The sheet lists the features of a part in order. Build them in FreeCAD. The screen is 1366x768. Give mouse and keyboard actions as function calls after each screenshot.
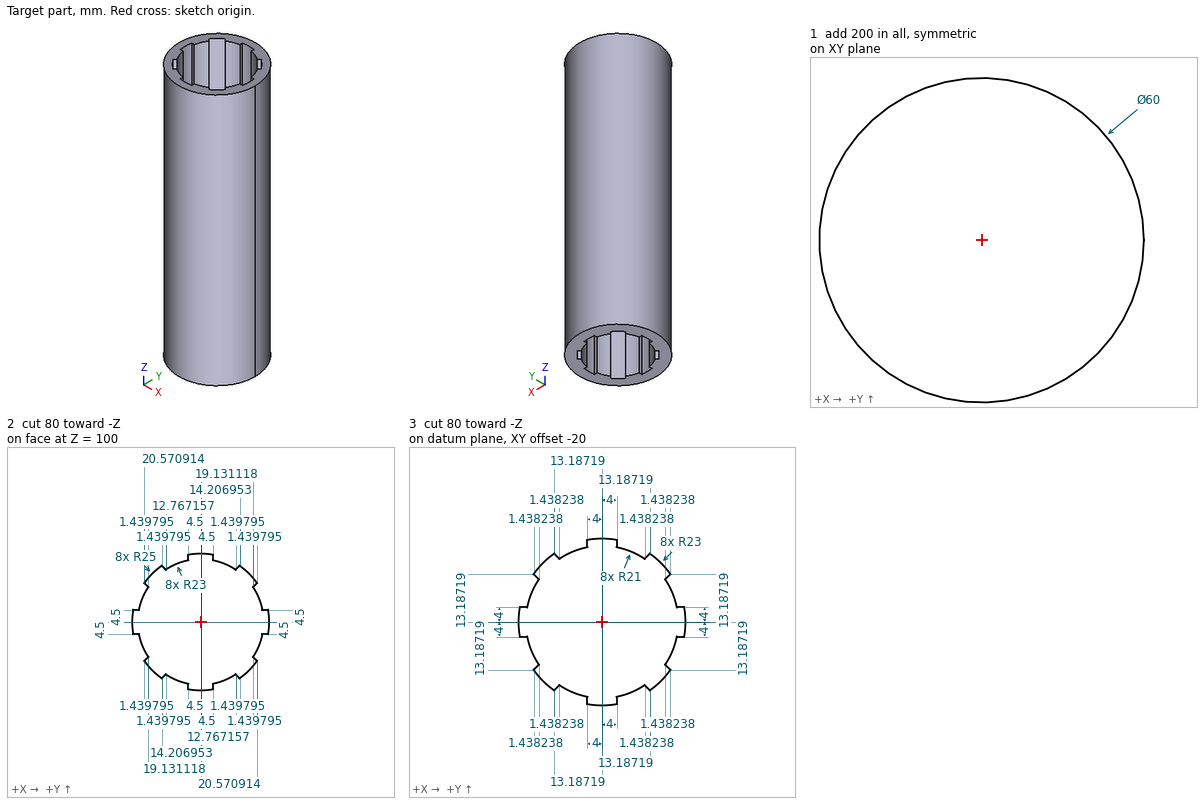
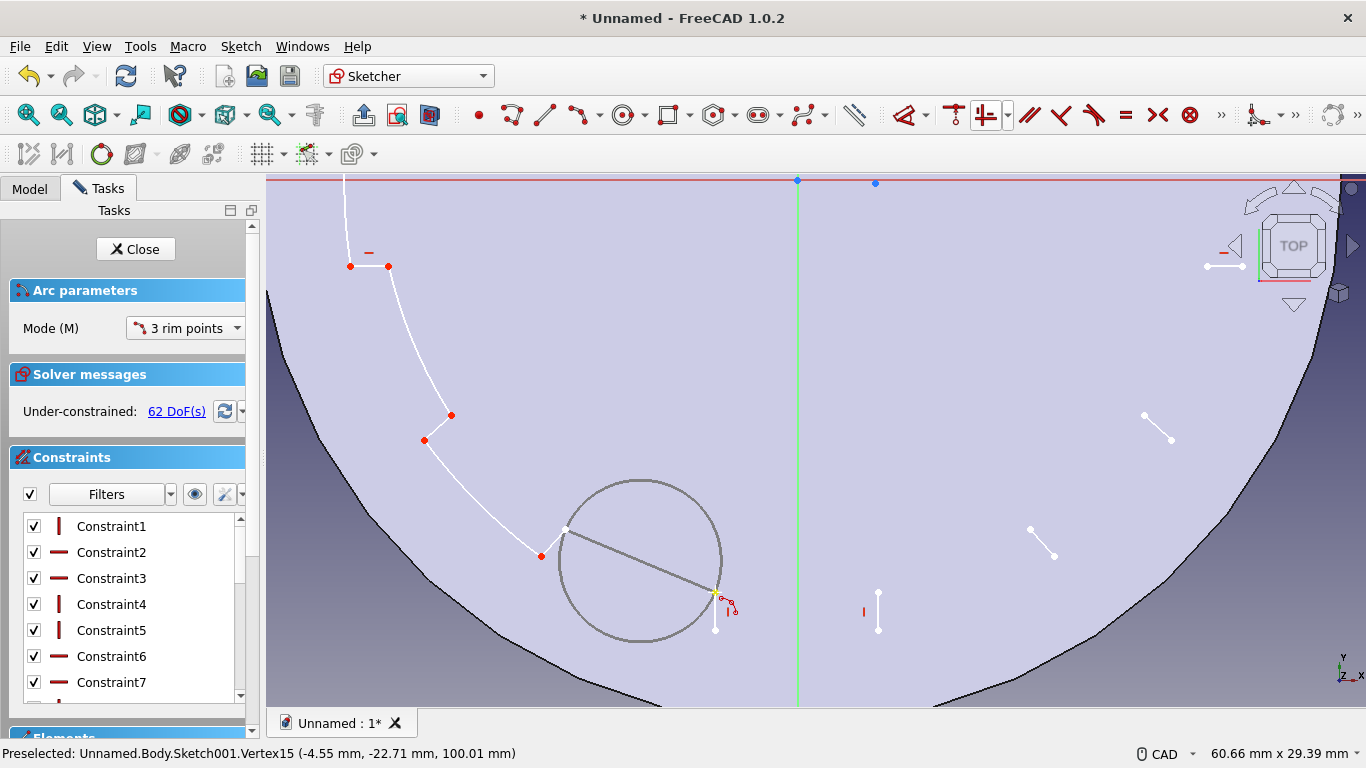
scroll(638, 566, up, 4)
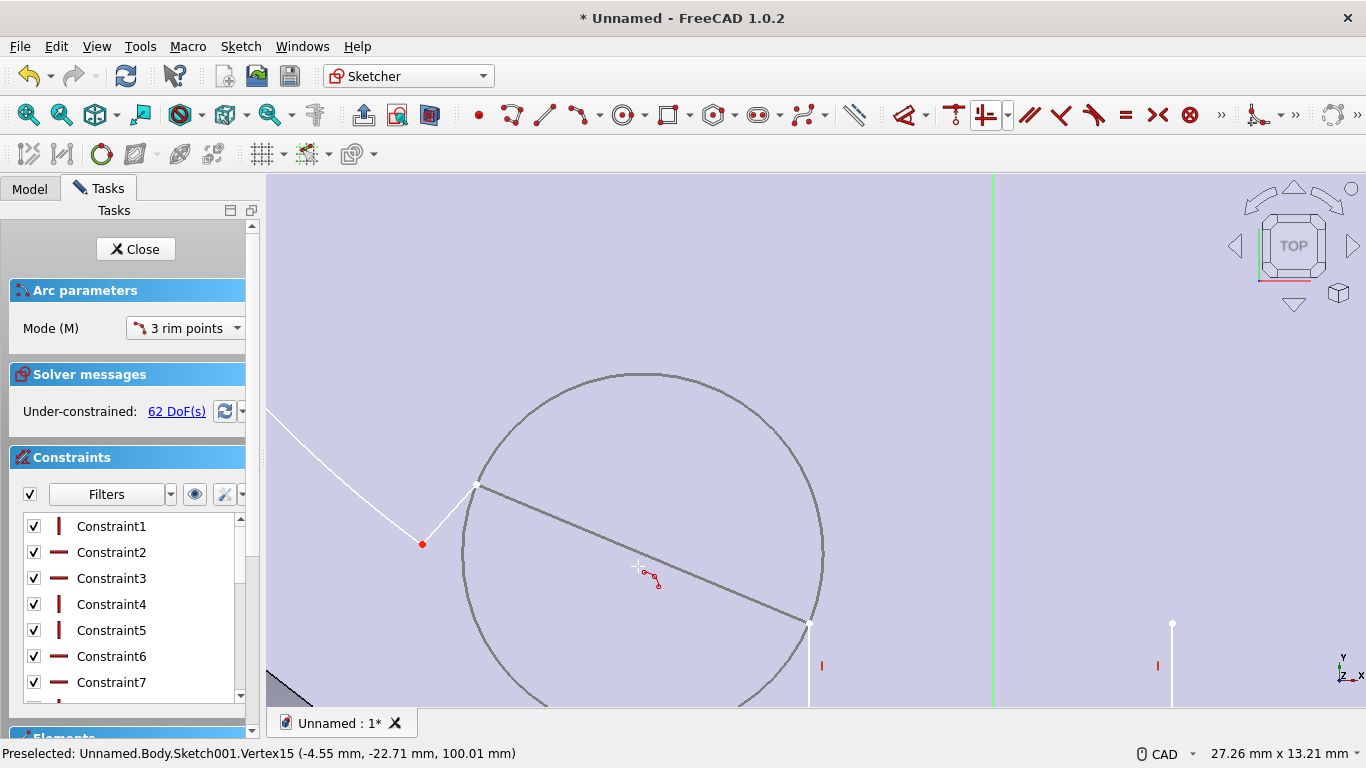
click(638, 565)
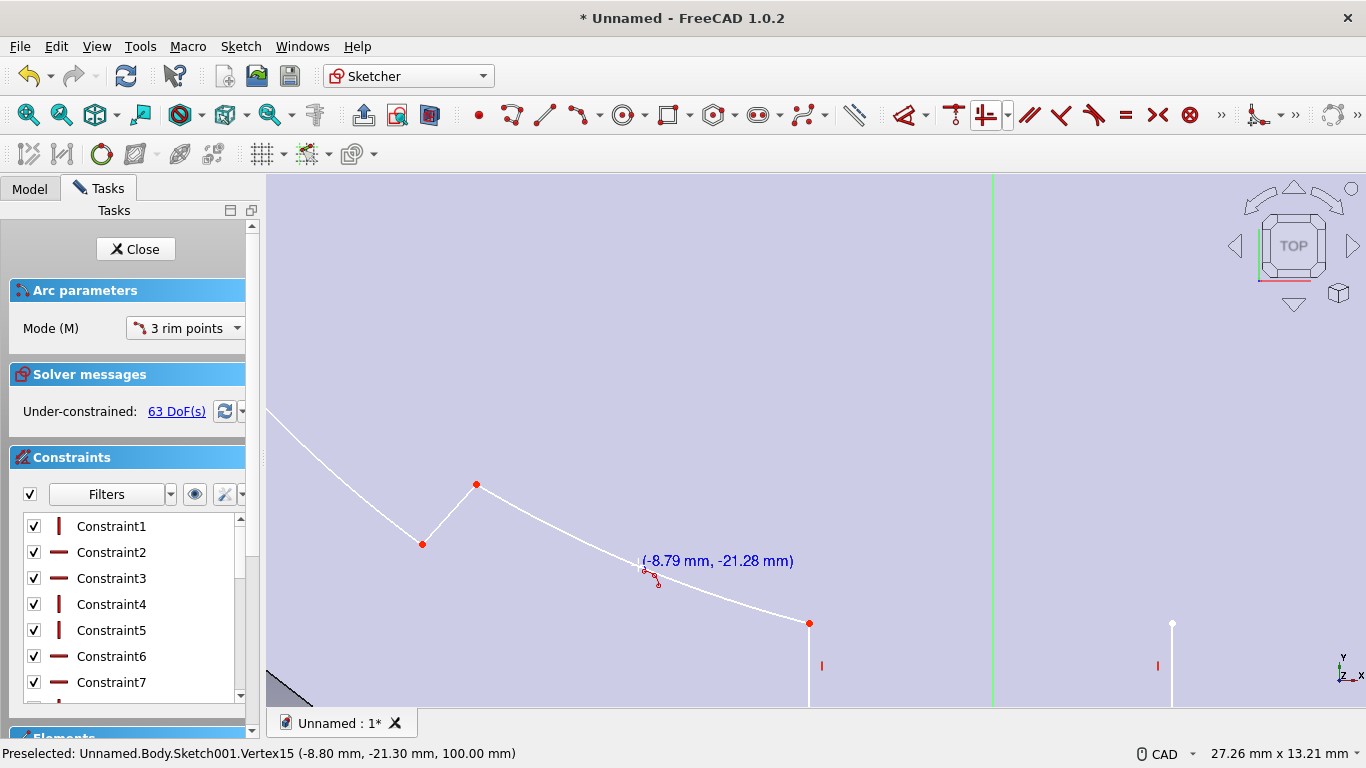
scroll(699, 586, down, 9)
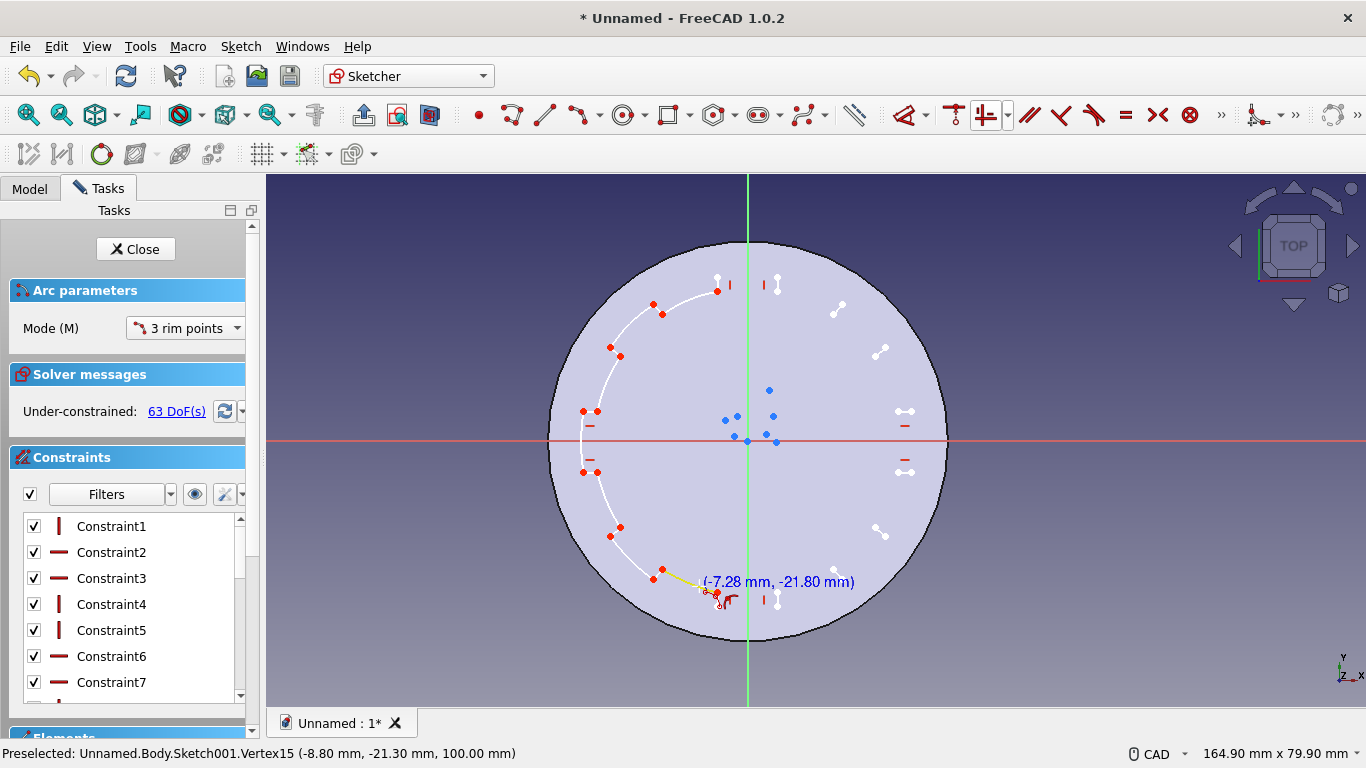
scroll(718, 605, up, 5)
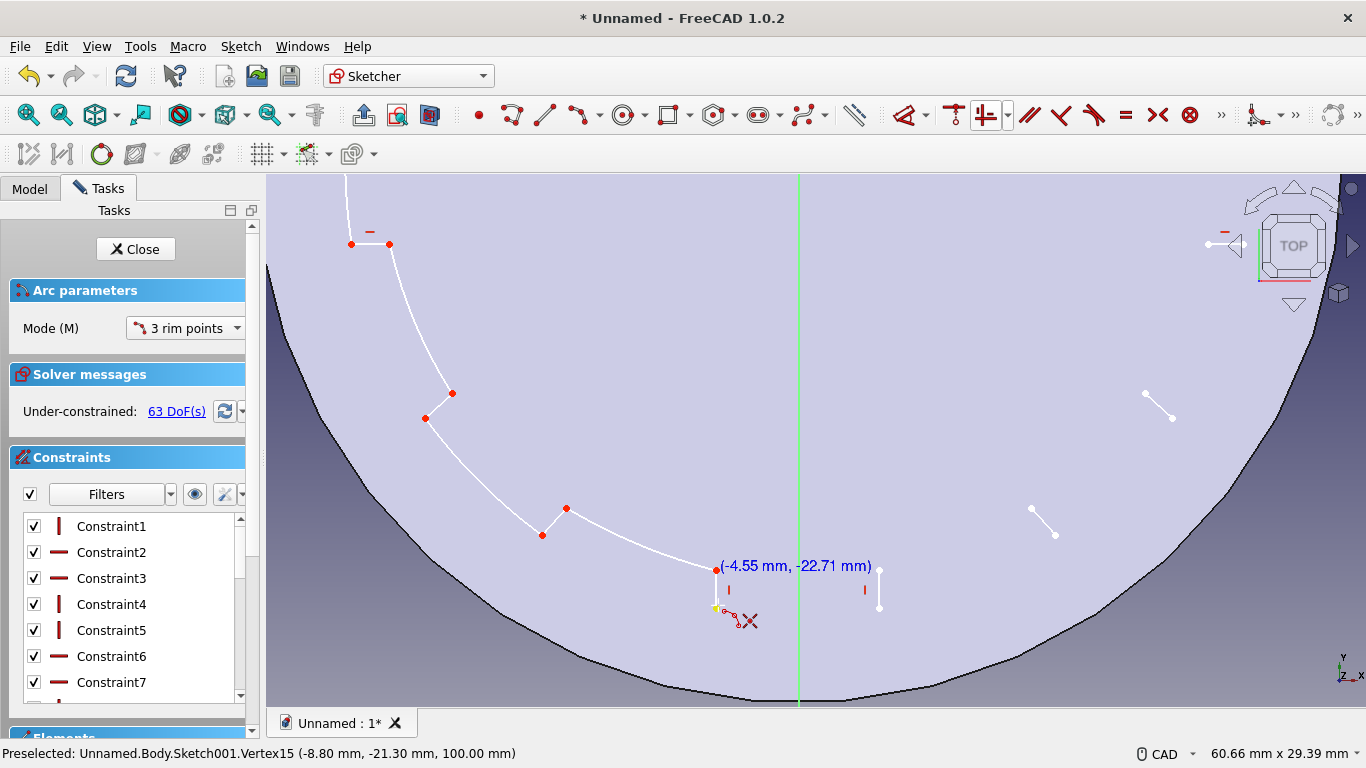
click(716, 609)
click(879, 609)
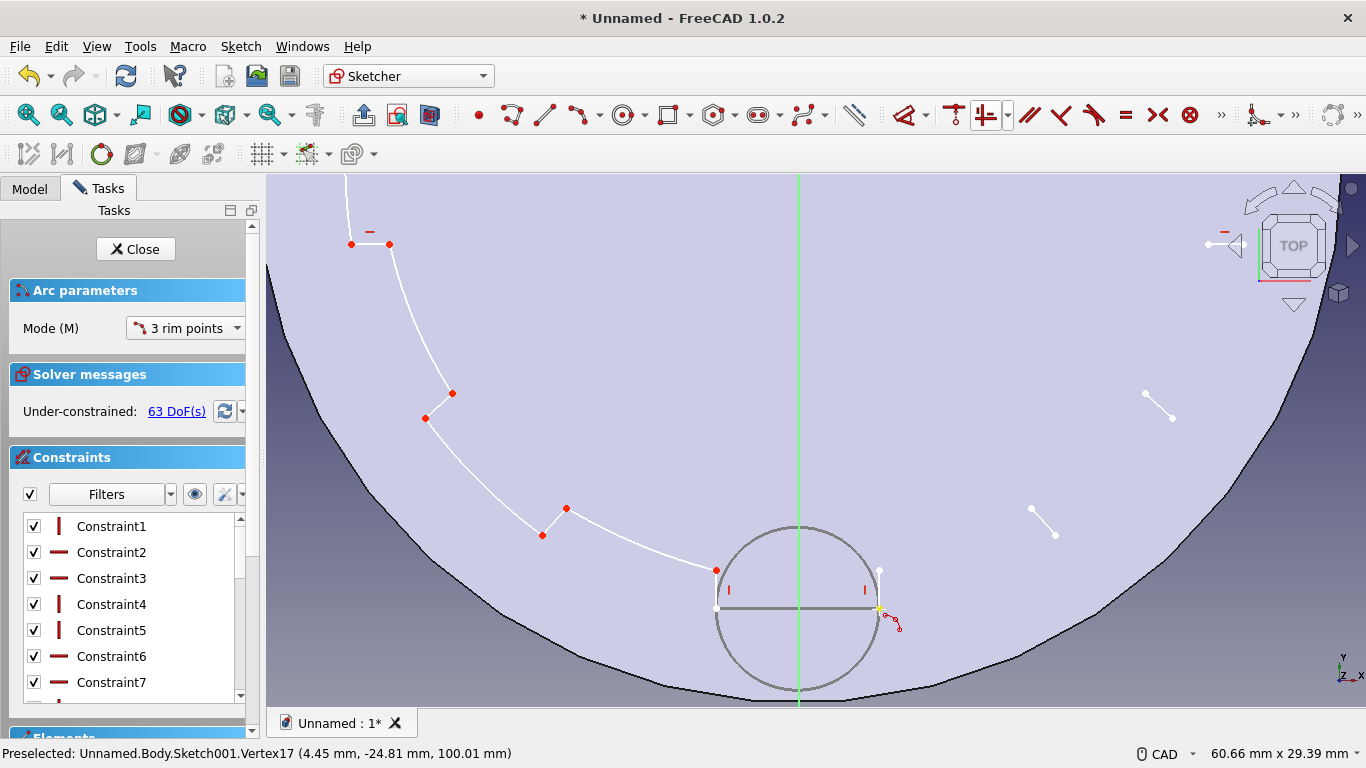
scroll(782, 612, up, 5)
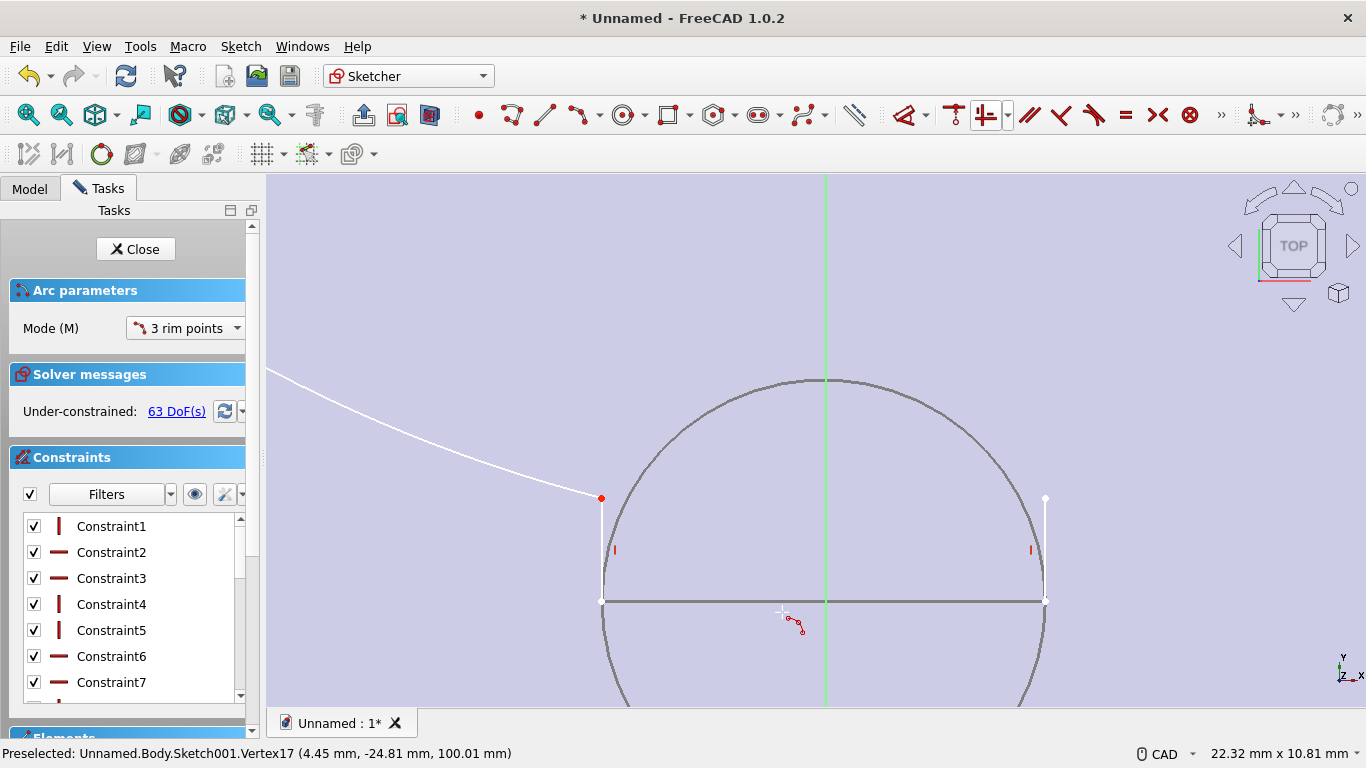
click(782, 610)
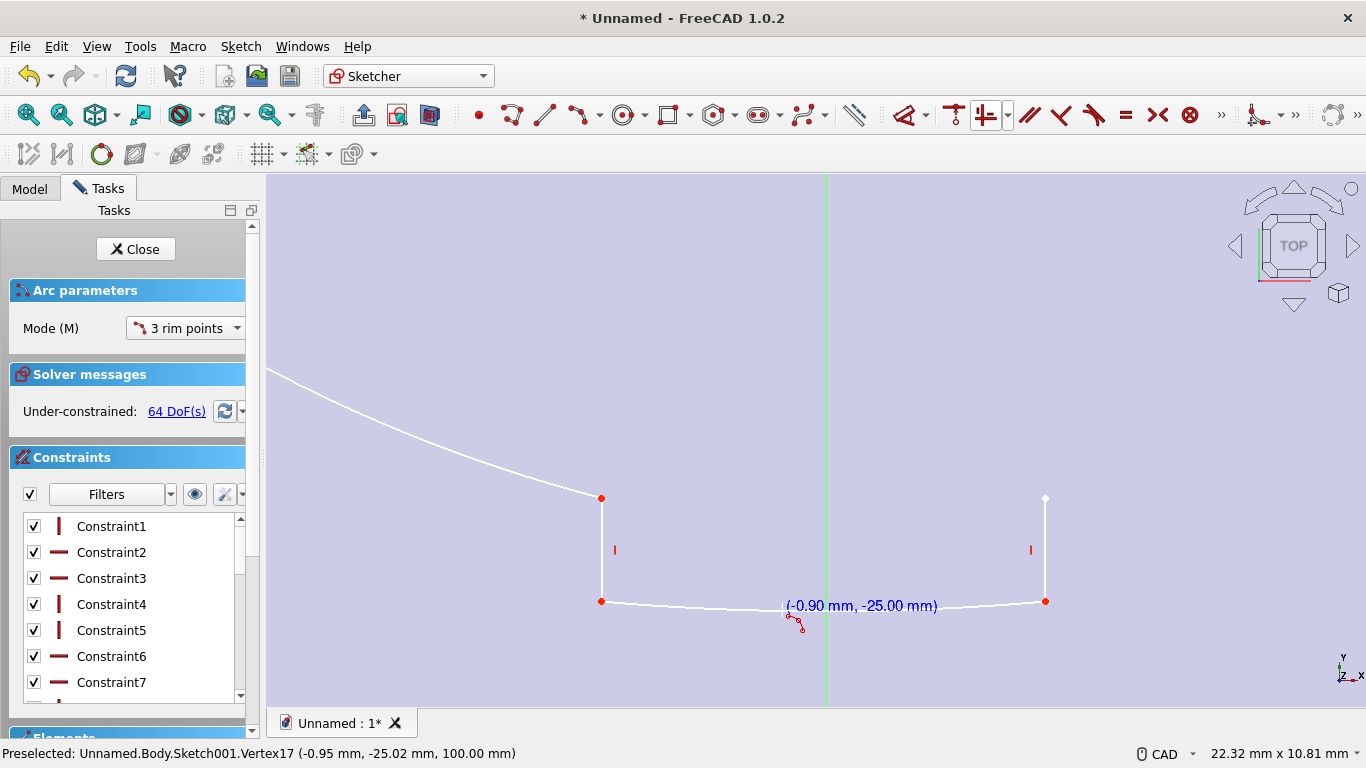
scroll(735, 607, down, 10)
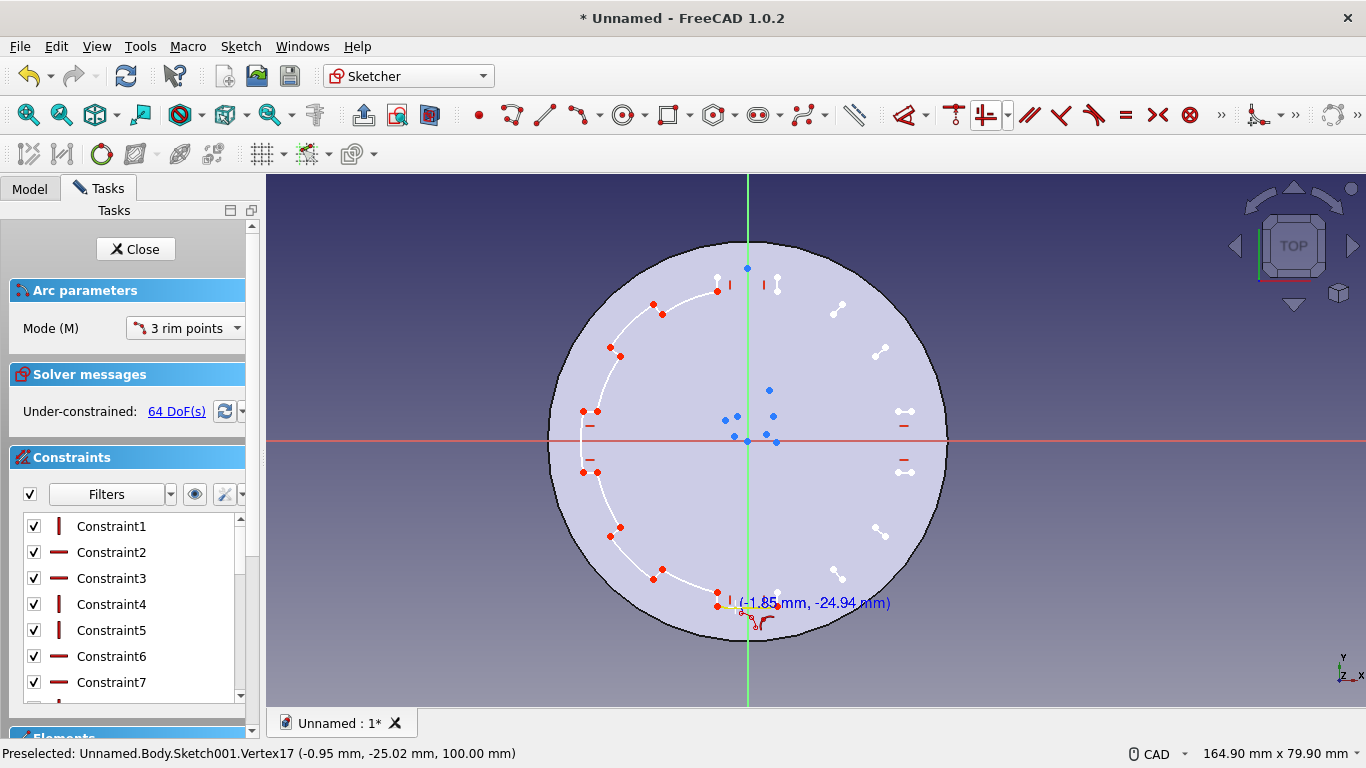
scroll(778, 592, up, 5)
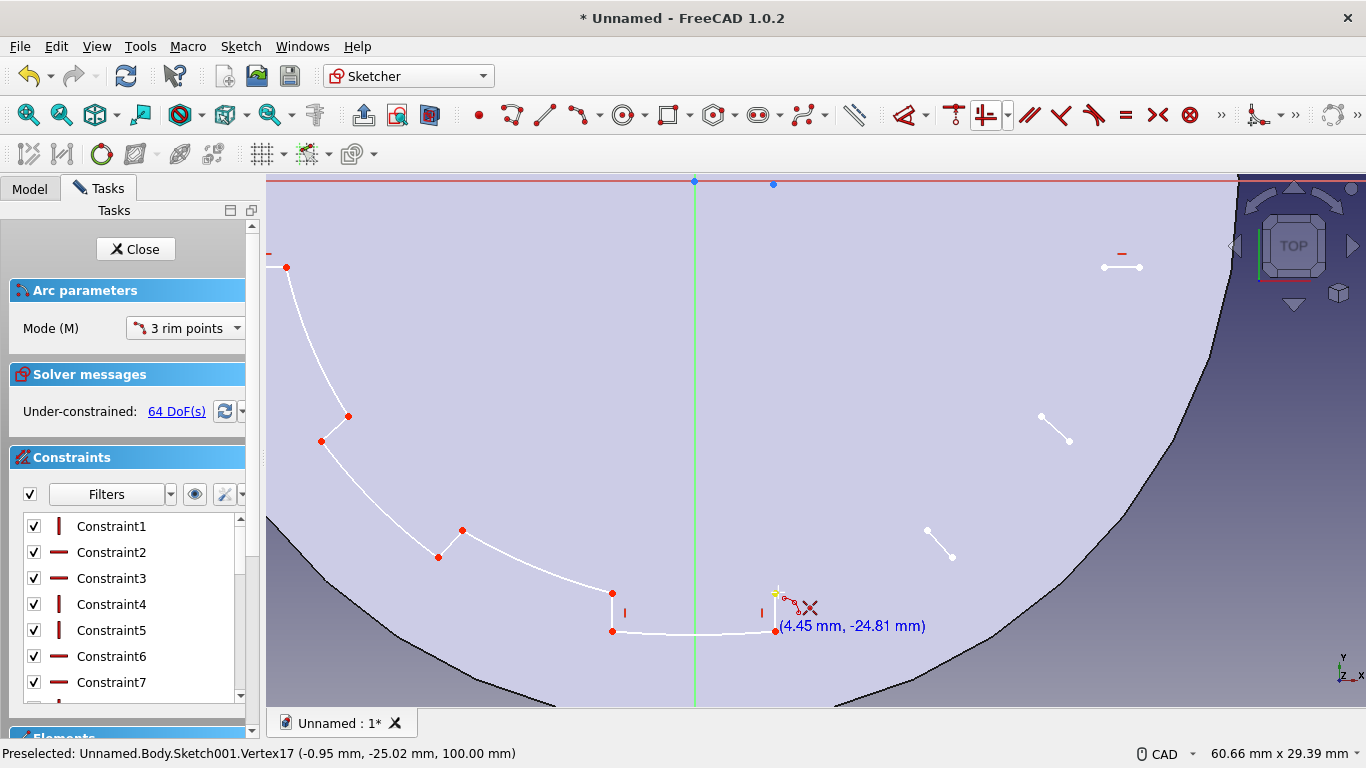
click(775, 593)
click(928, 531)